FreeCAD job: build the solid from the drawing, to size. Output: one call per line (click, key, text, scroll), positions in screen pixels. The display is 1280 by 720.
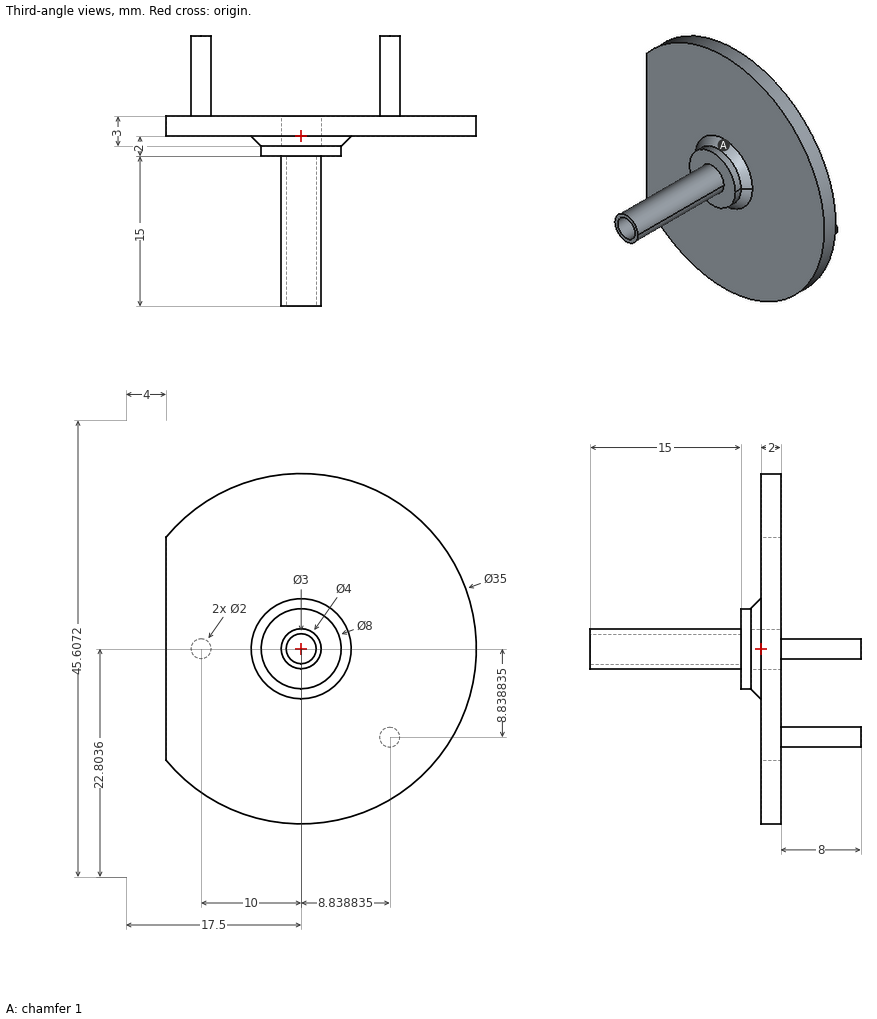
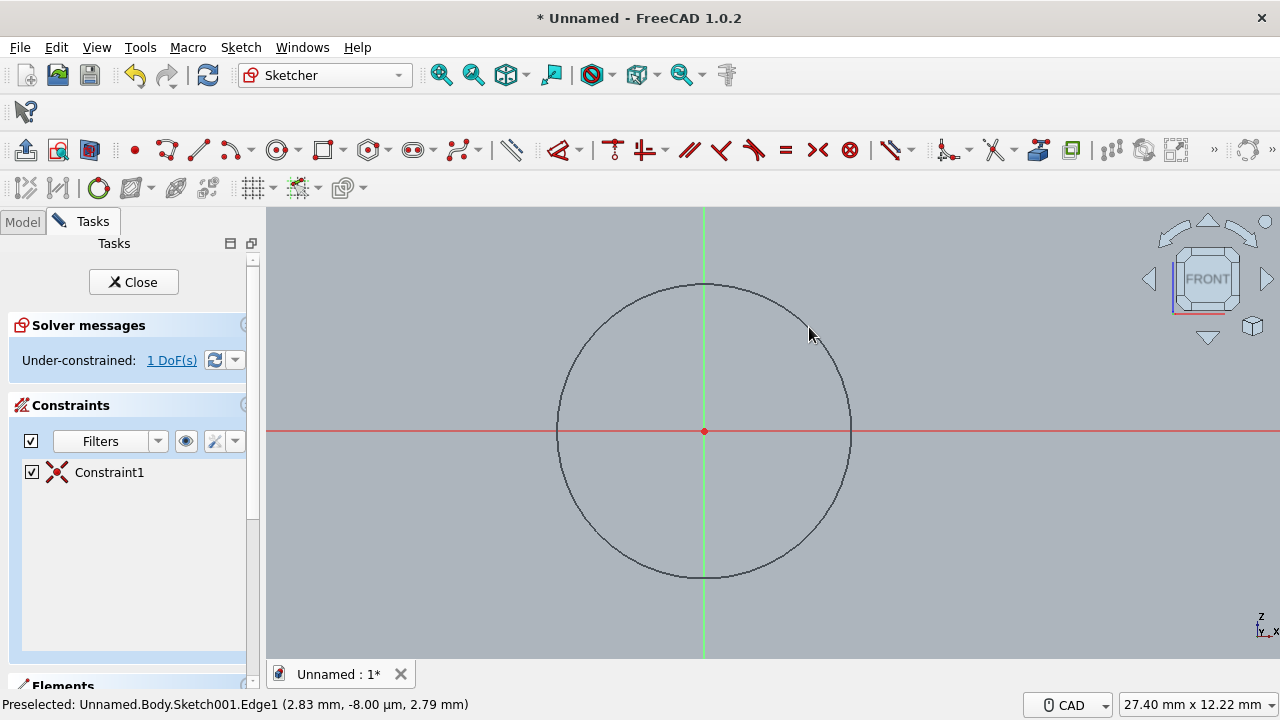
click(558, 150)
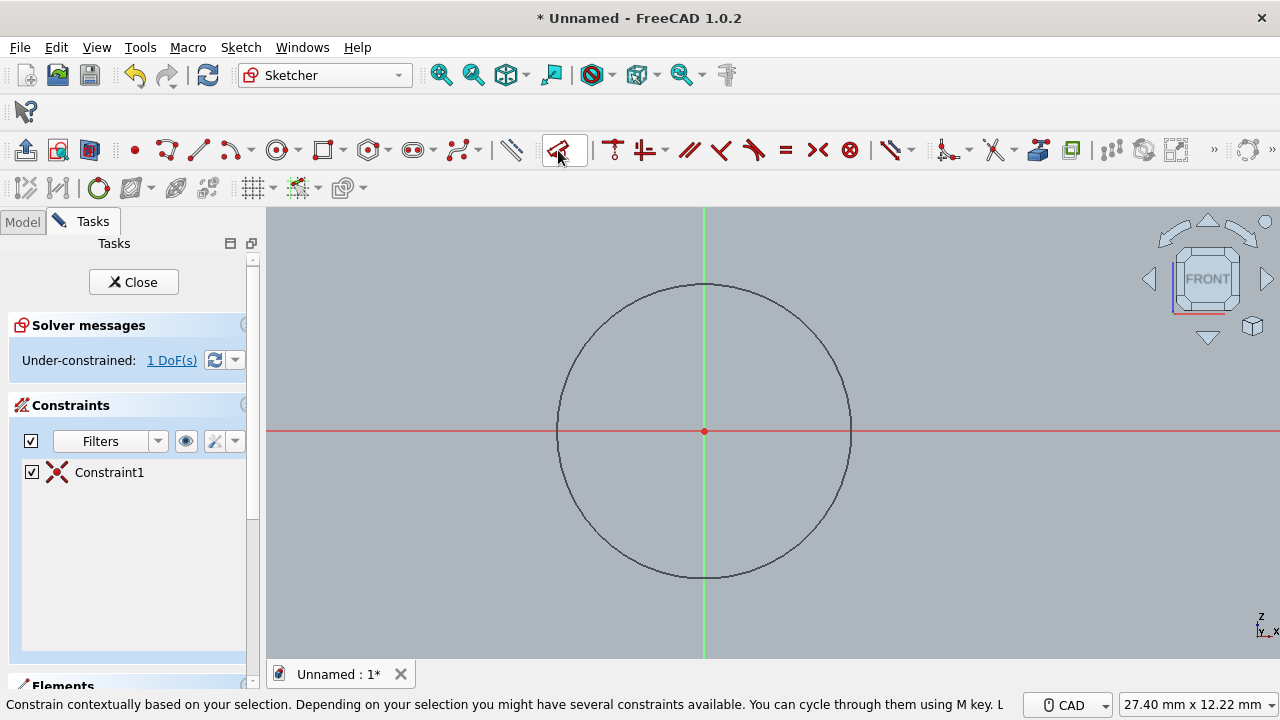
click(808, 327)
click(831, 304)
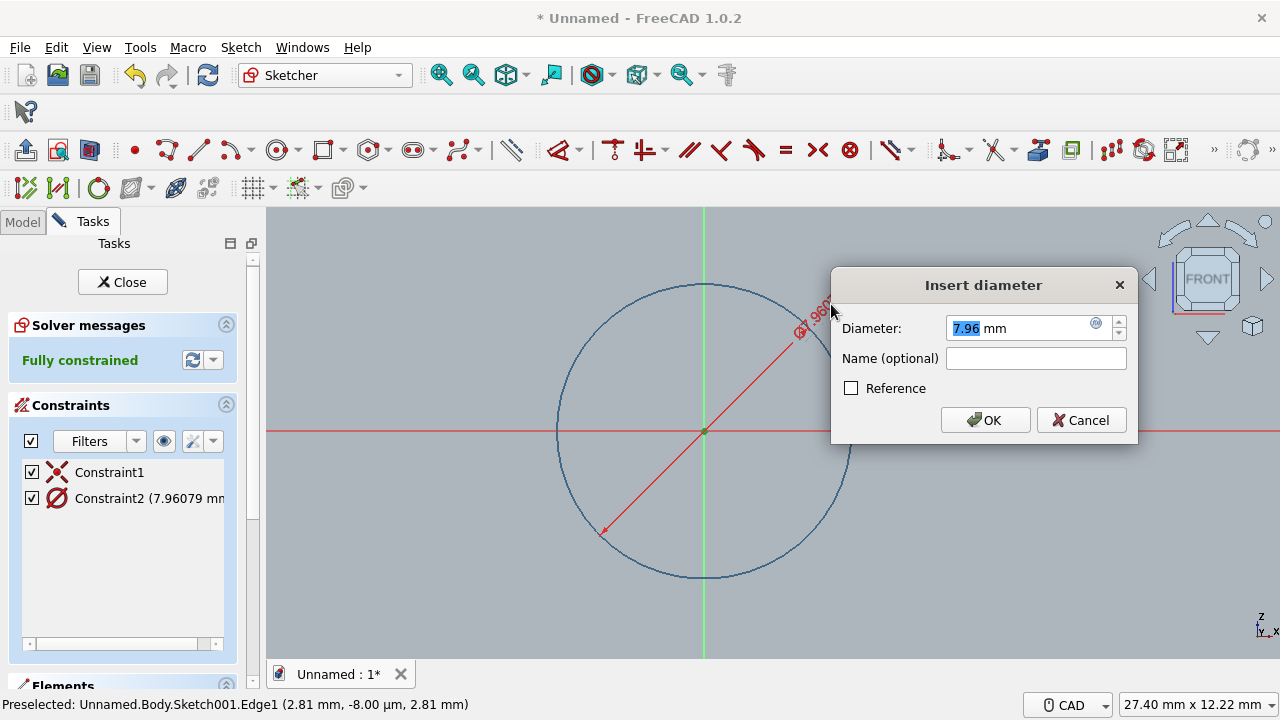
text(8)
key(Return)
key(Escape)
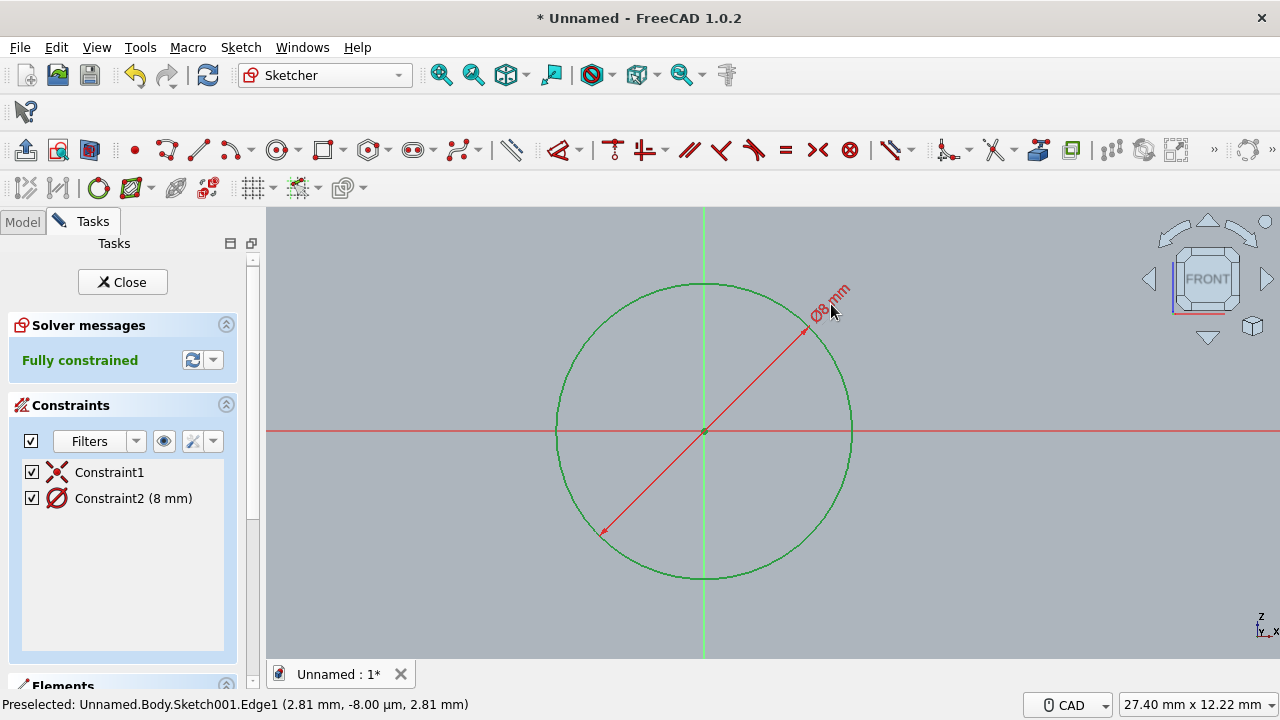
click(123, 282)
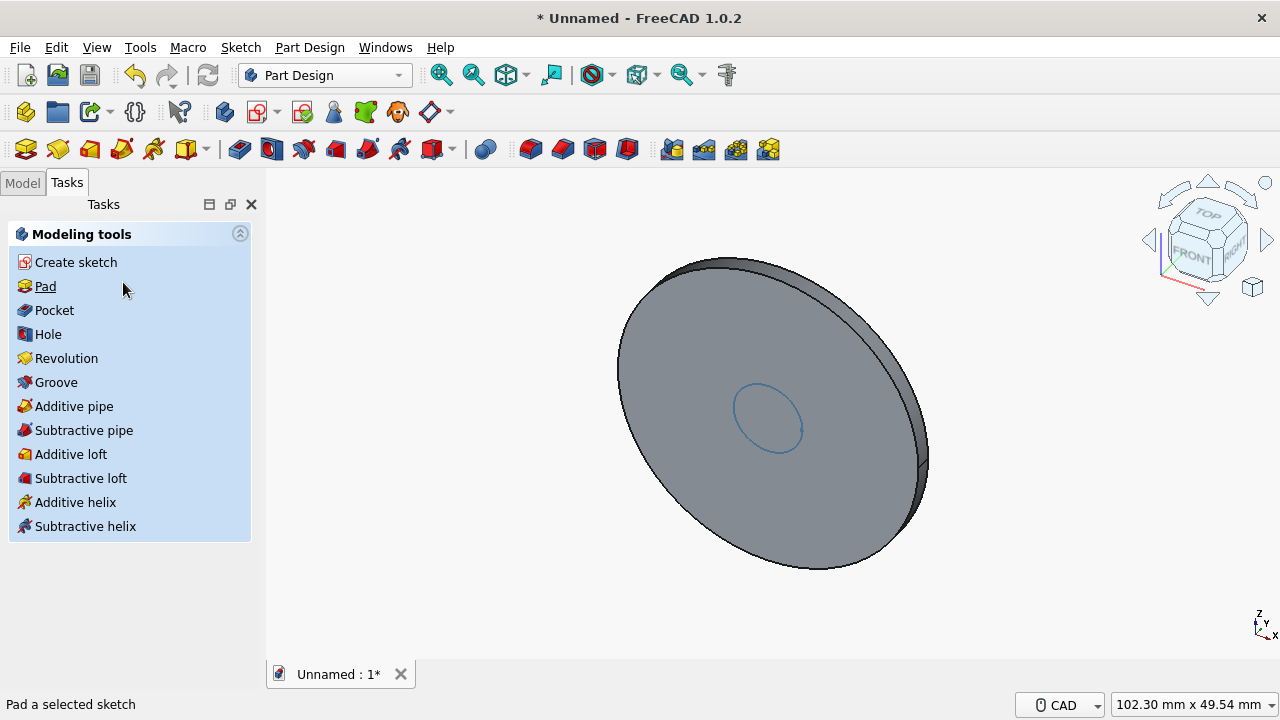
click(26, 150)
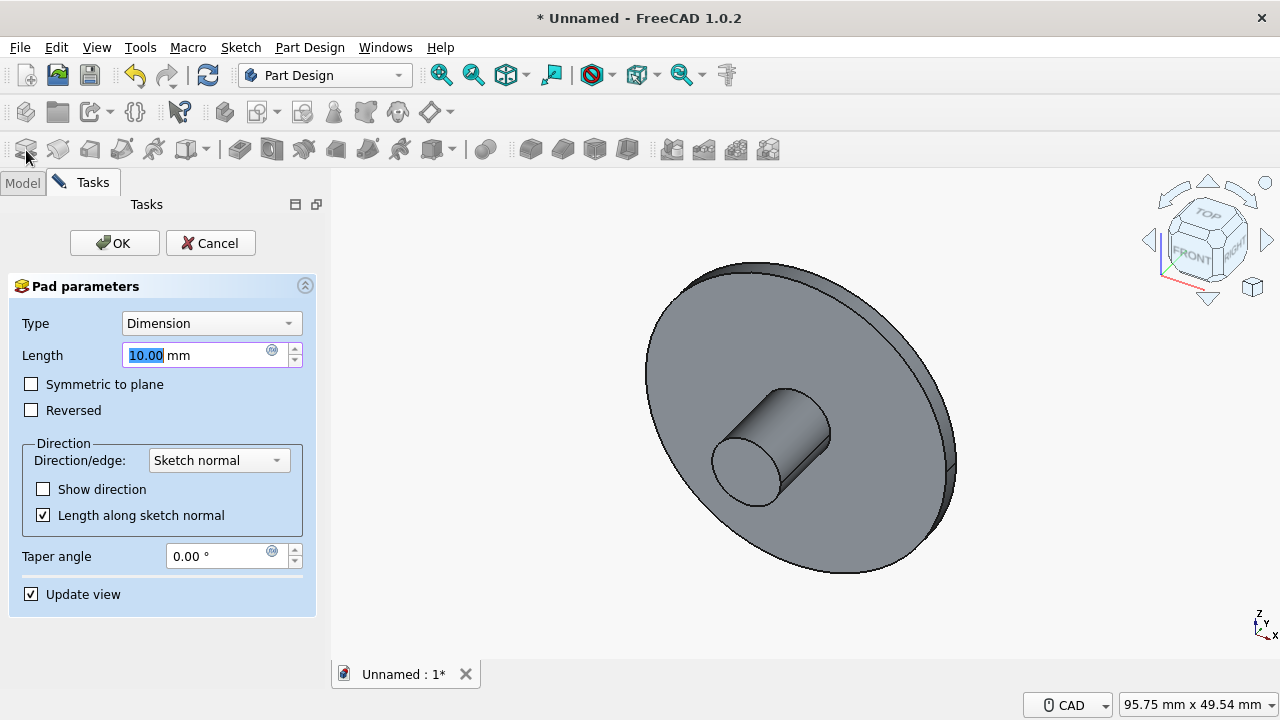
text(2)
key(Tab)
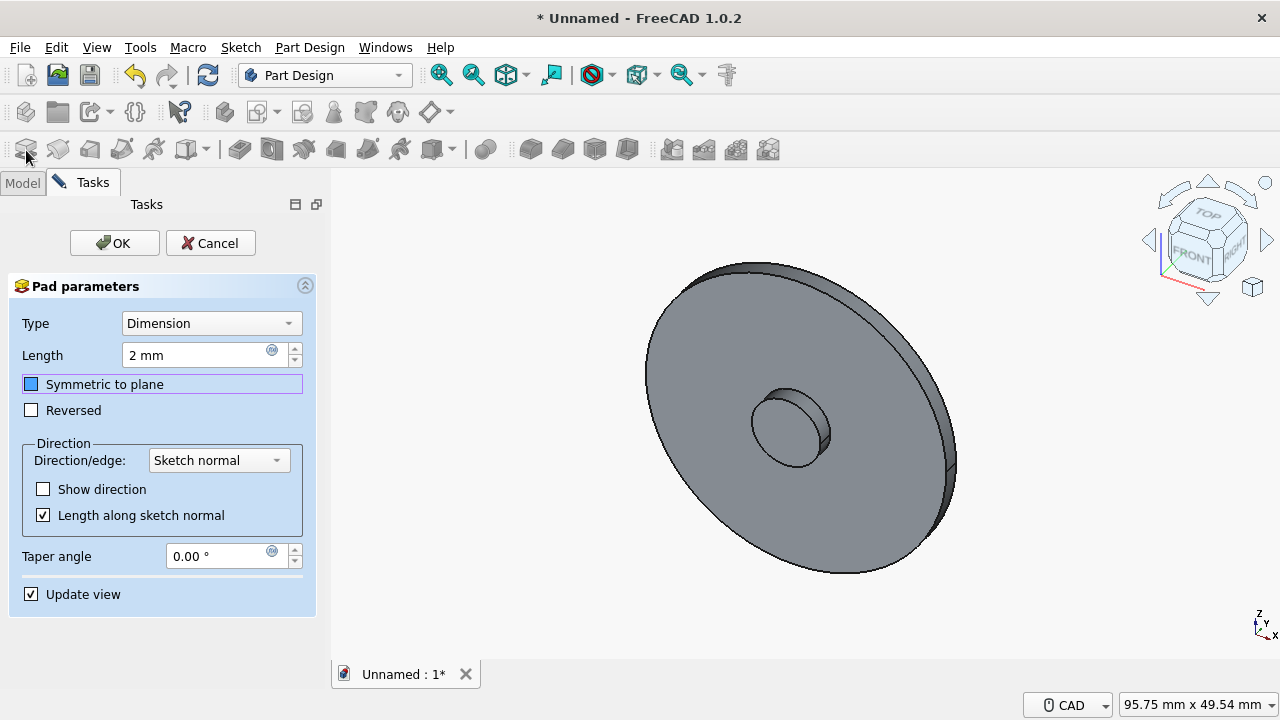
click(115, 243)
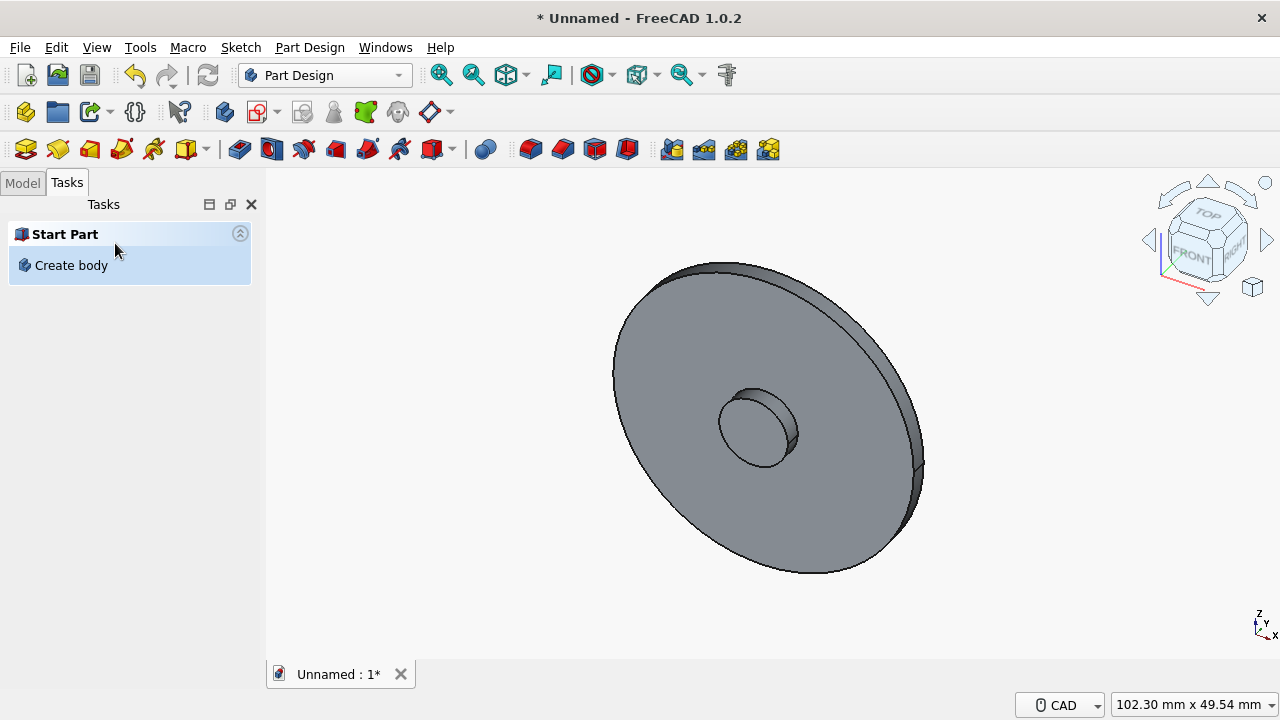
key(0)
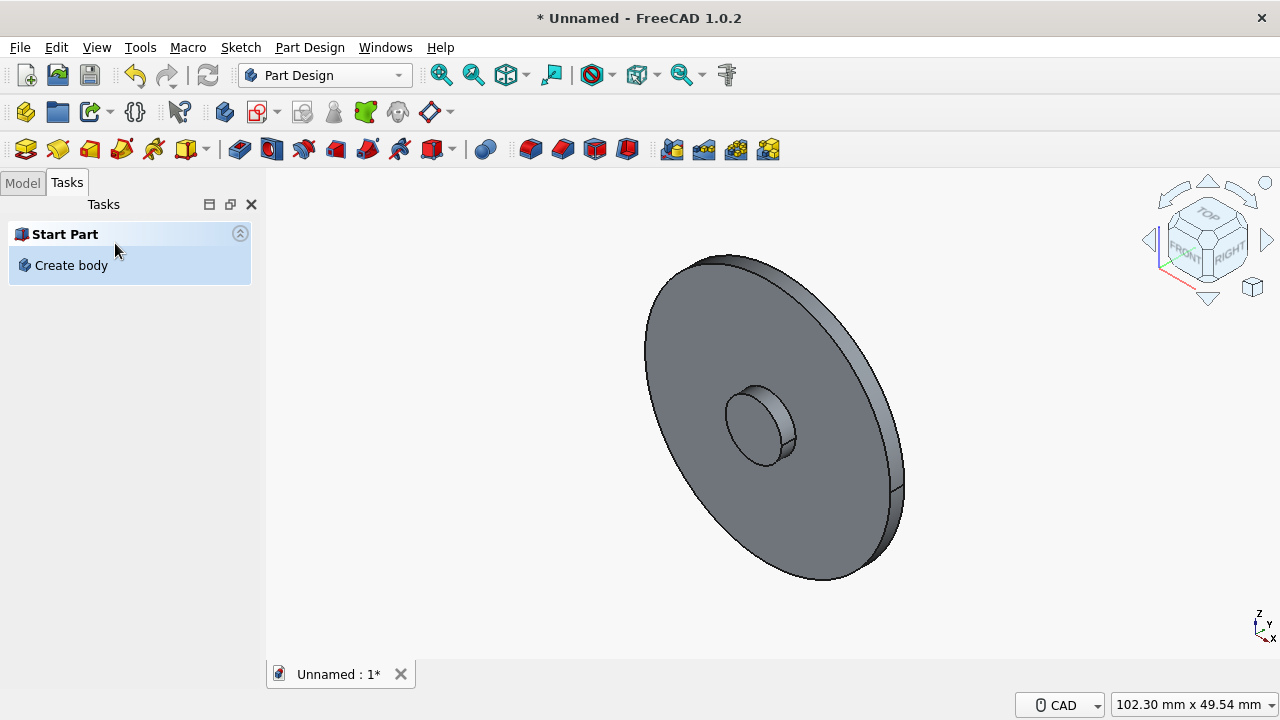
key(2)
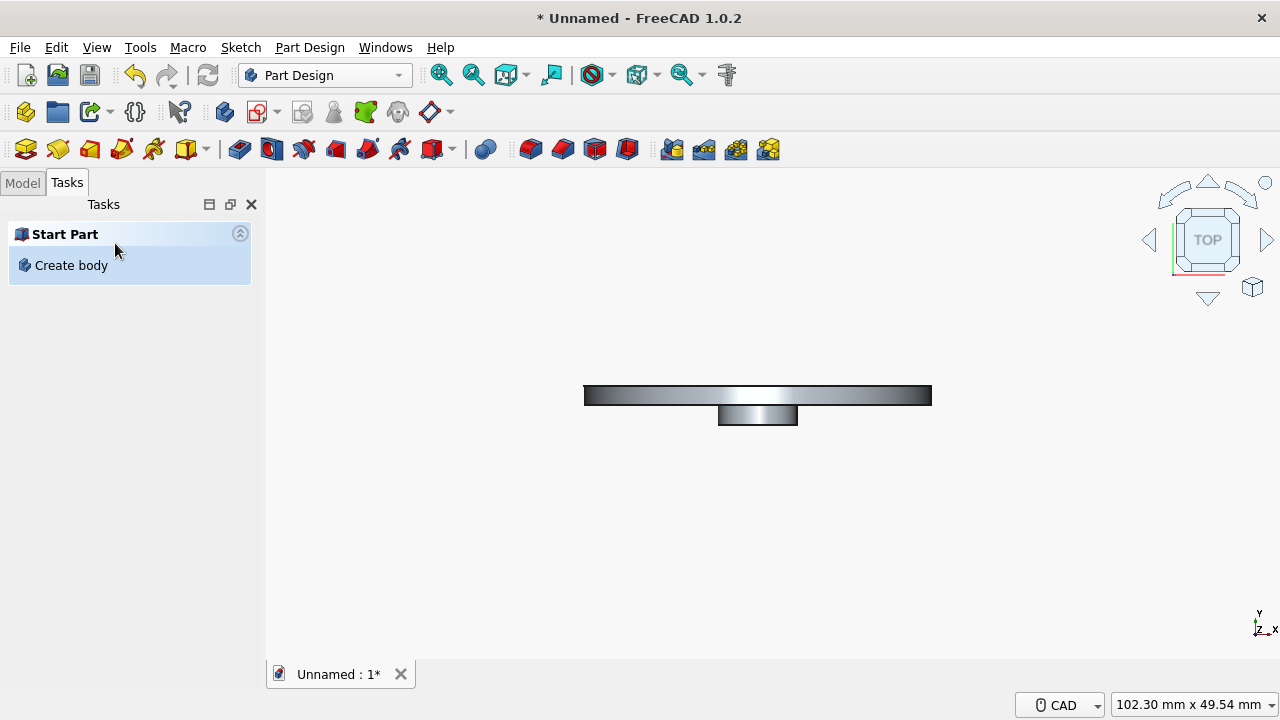
click(442, 76)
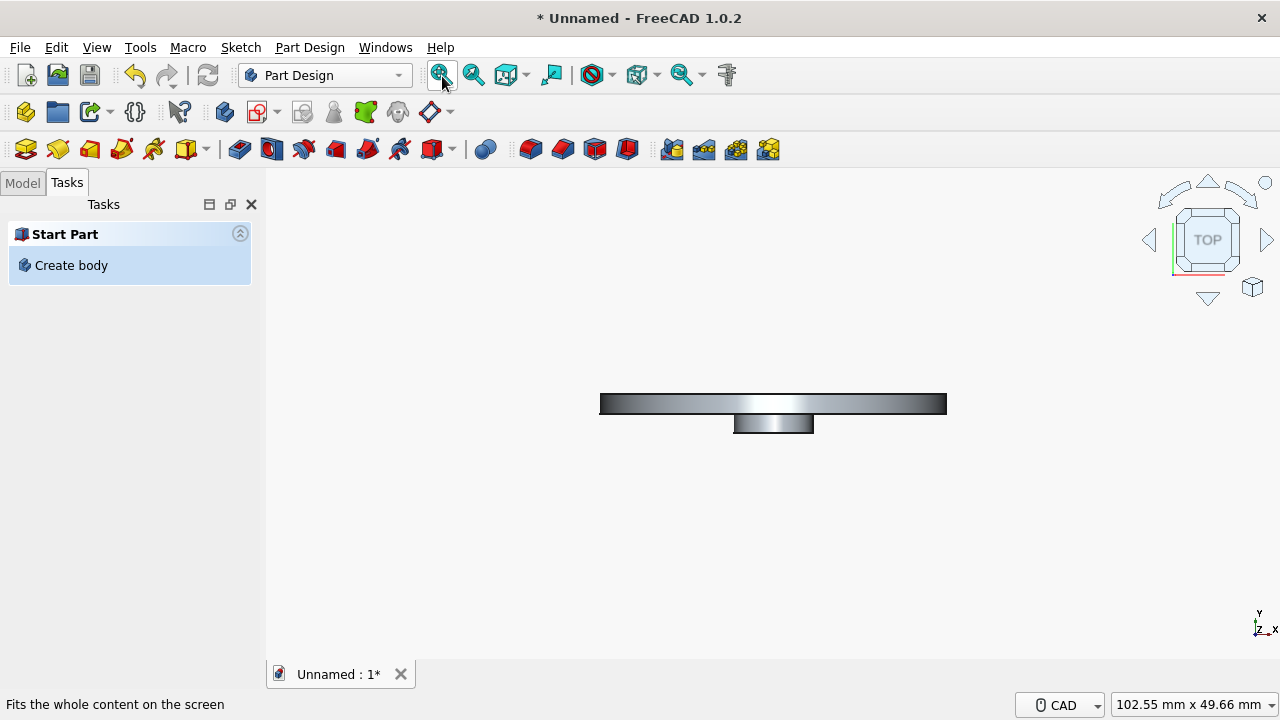
key(1)